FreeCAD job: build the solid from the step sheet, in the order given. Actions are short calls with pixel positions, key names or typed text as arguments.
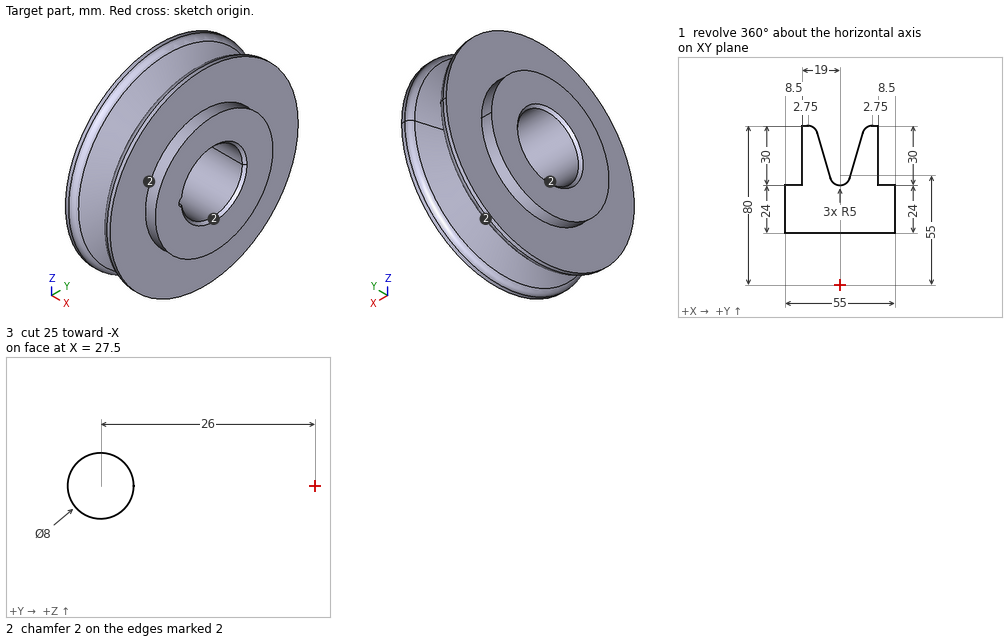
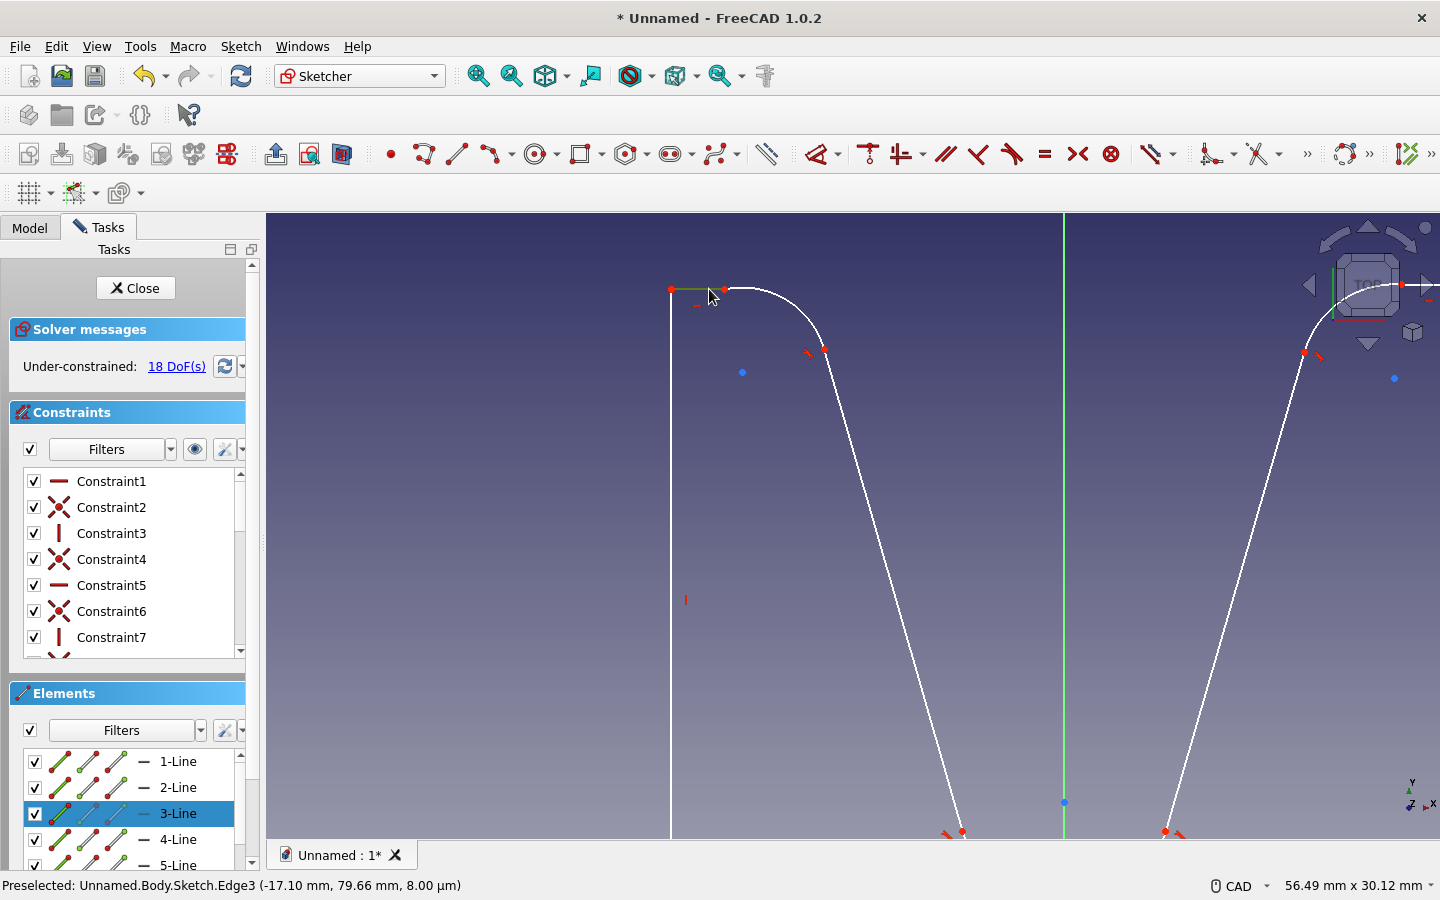
click(806, 316)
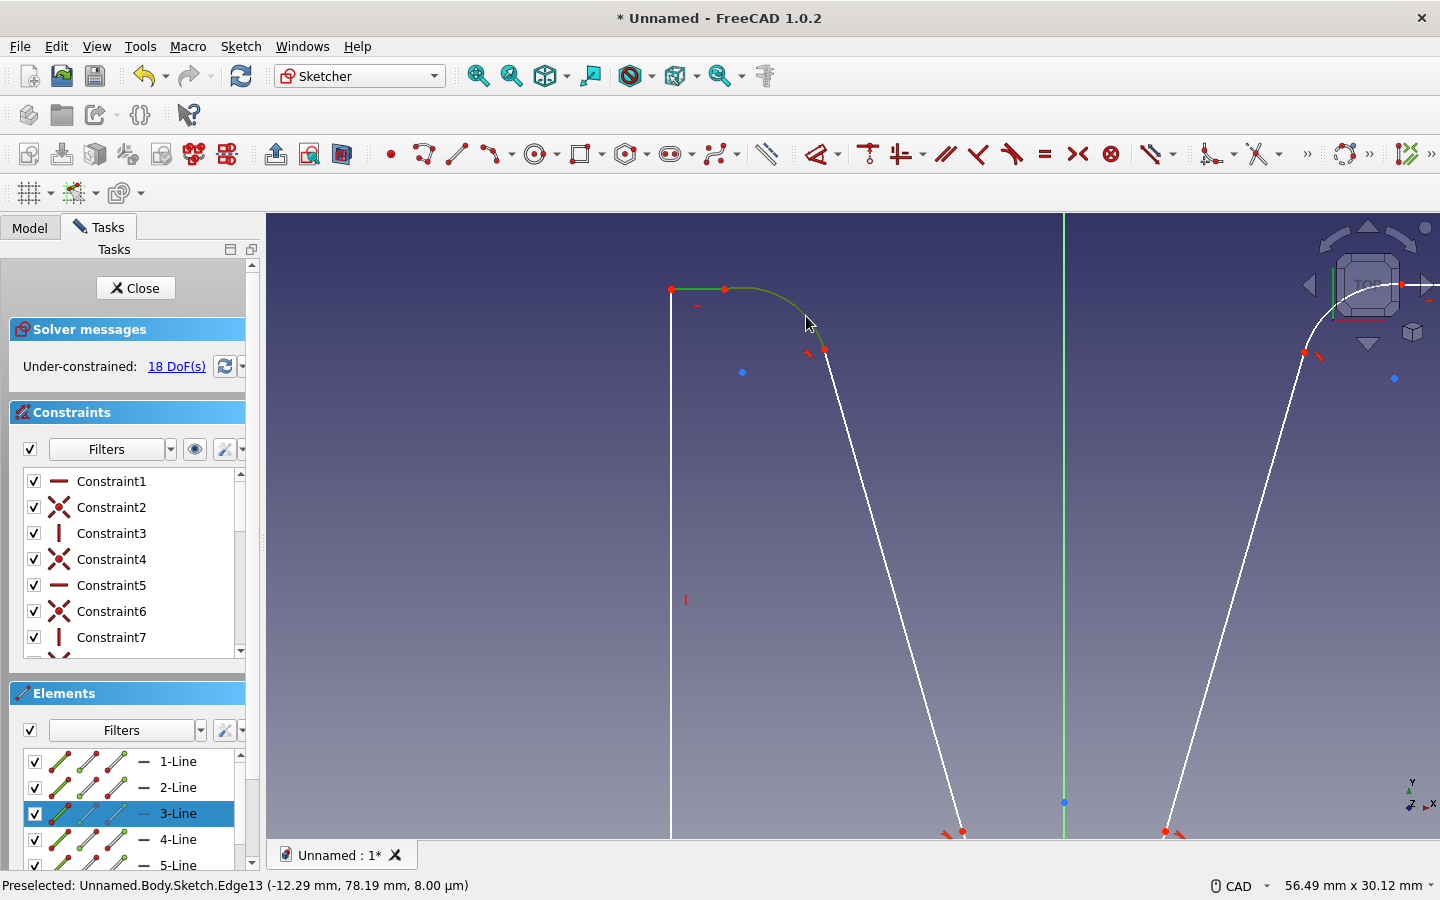
key(t)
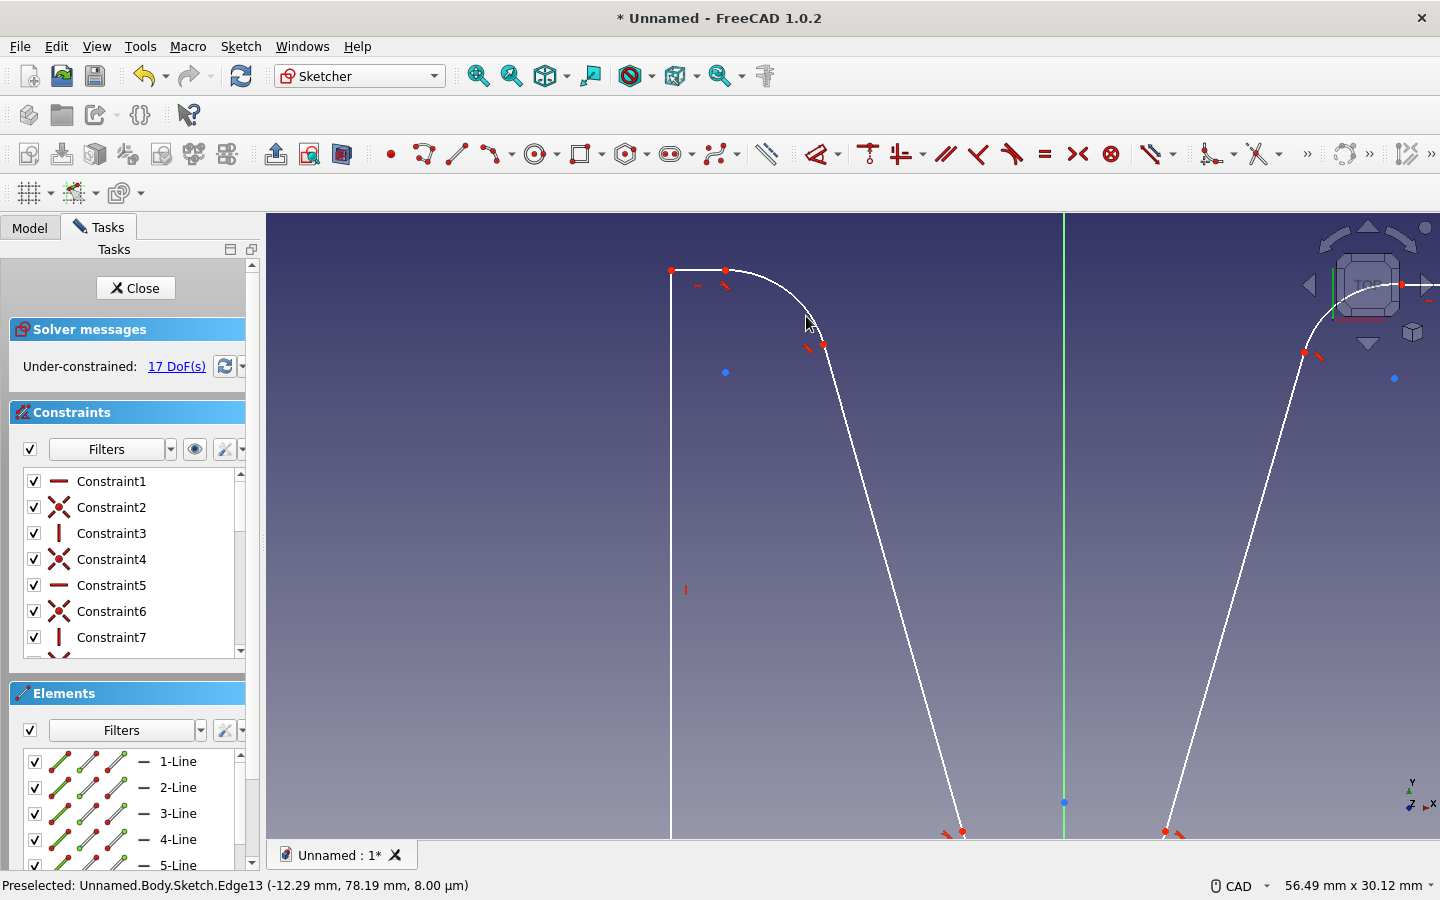
scroll(693, 334, down, 7)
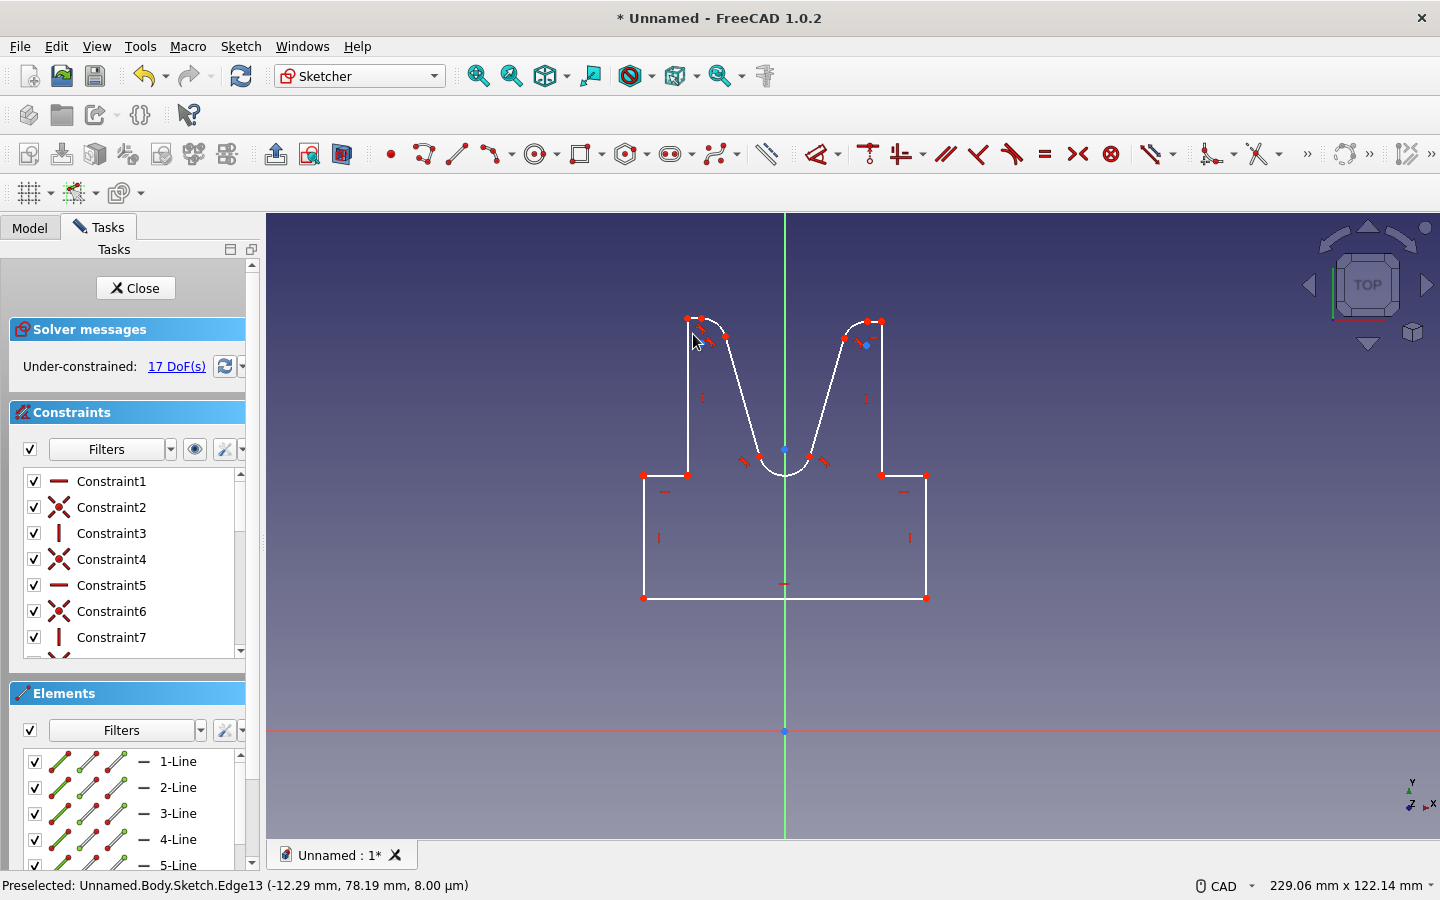
scroll(878, 322, up, 6)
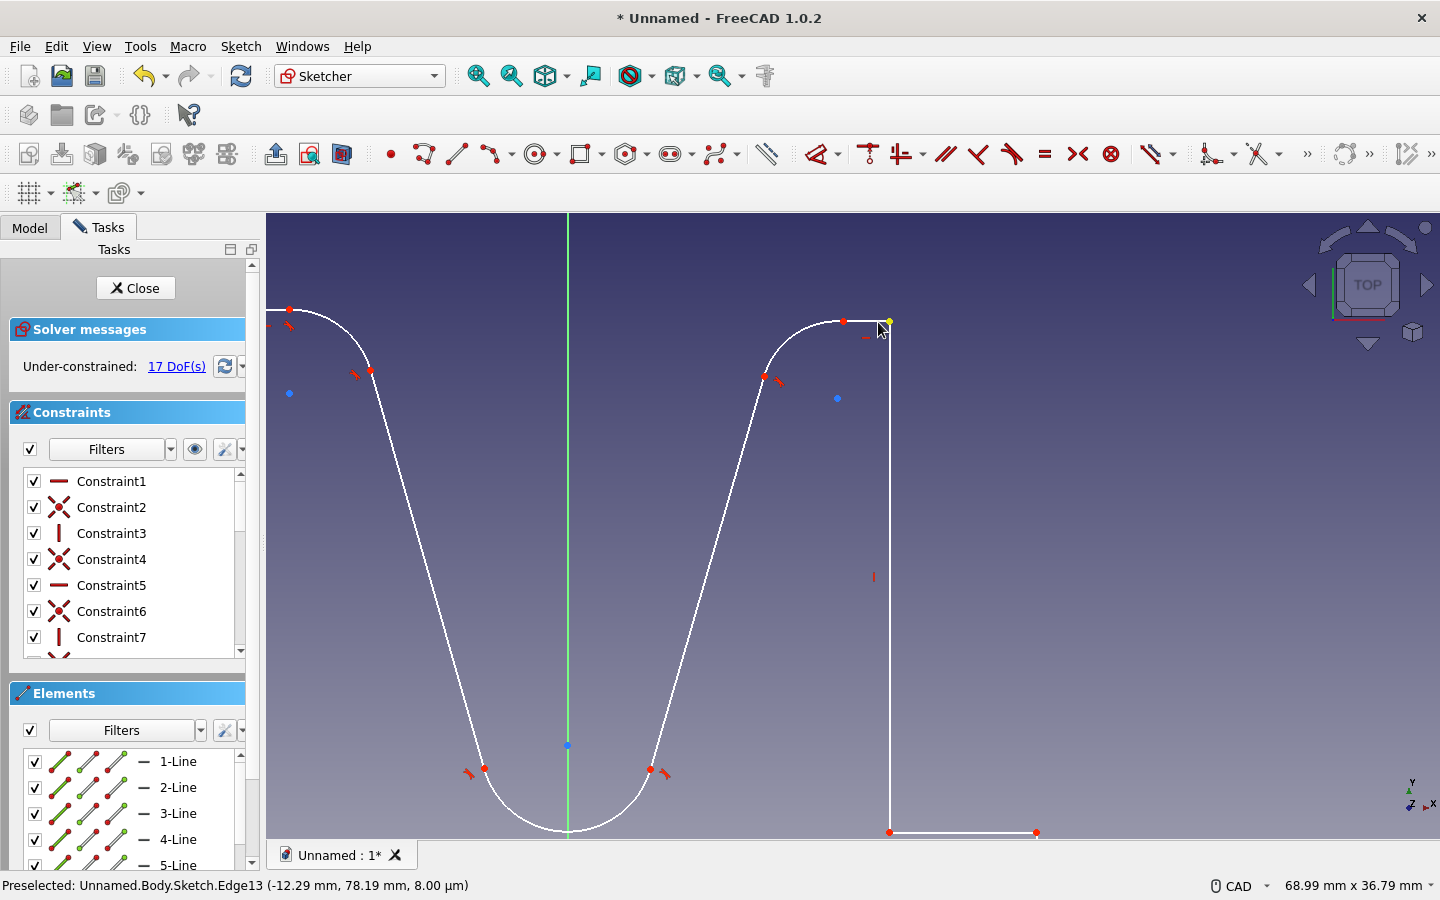
click(876, 321)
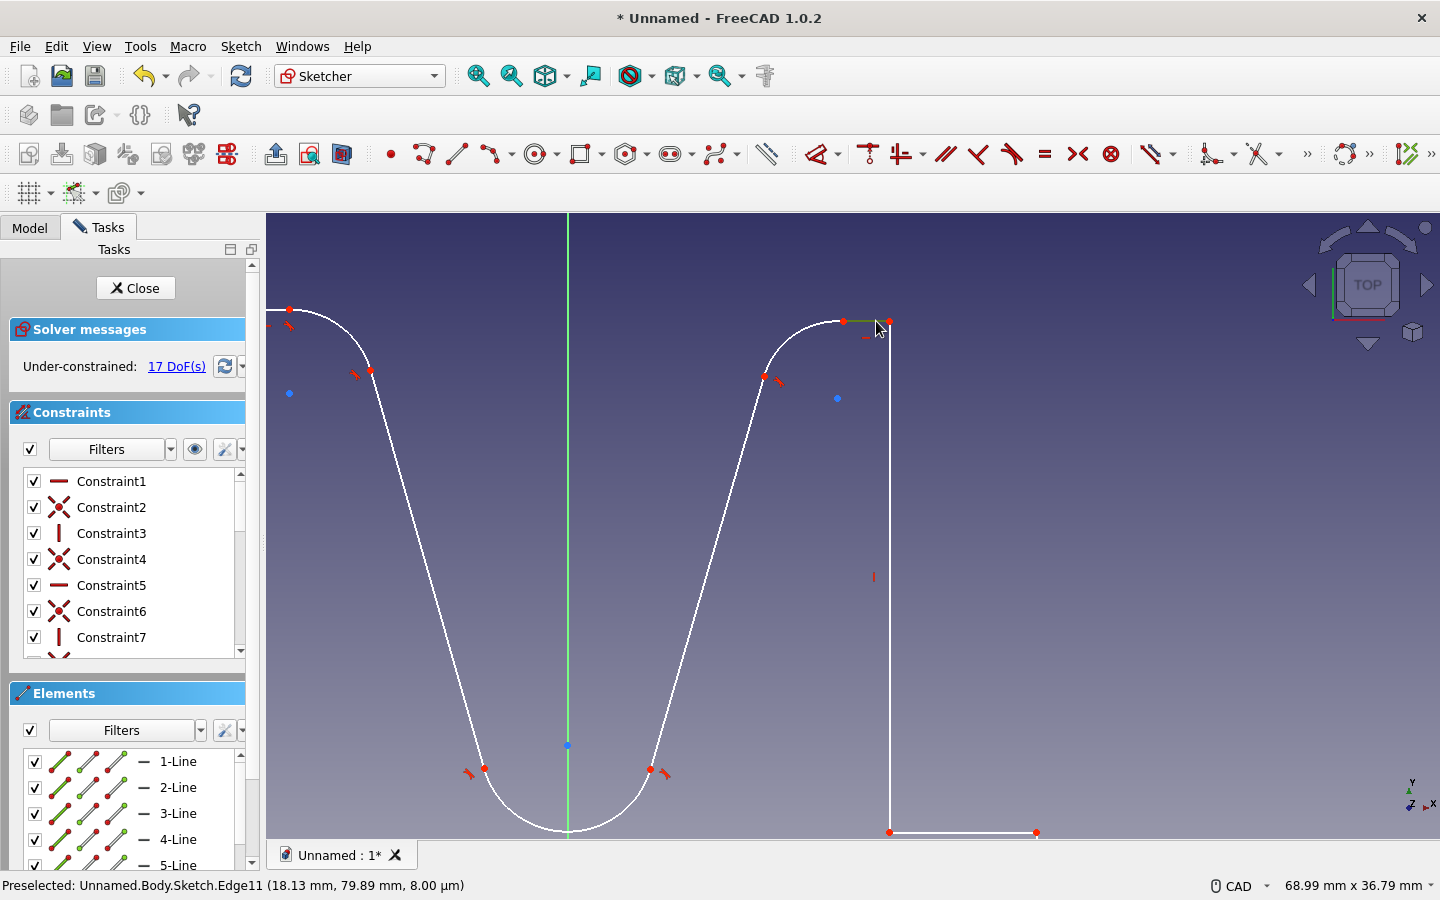
click(813, 326)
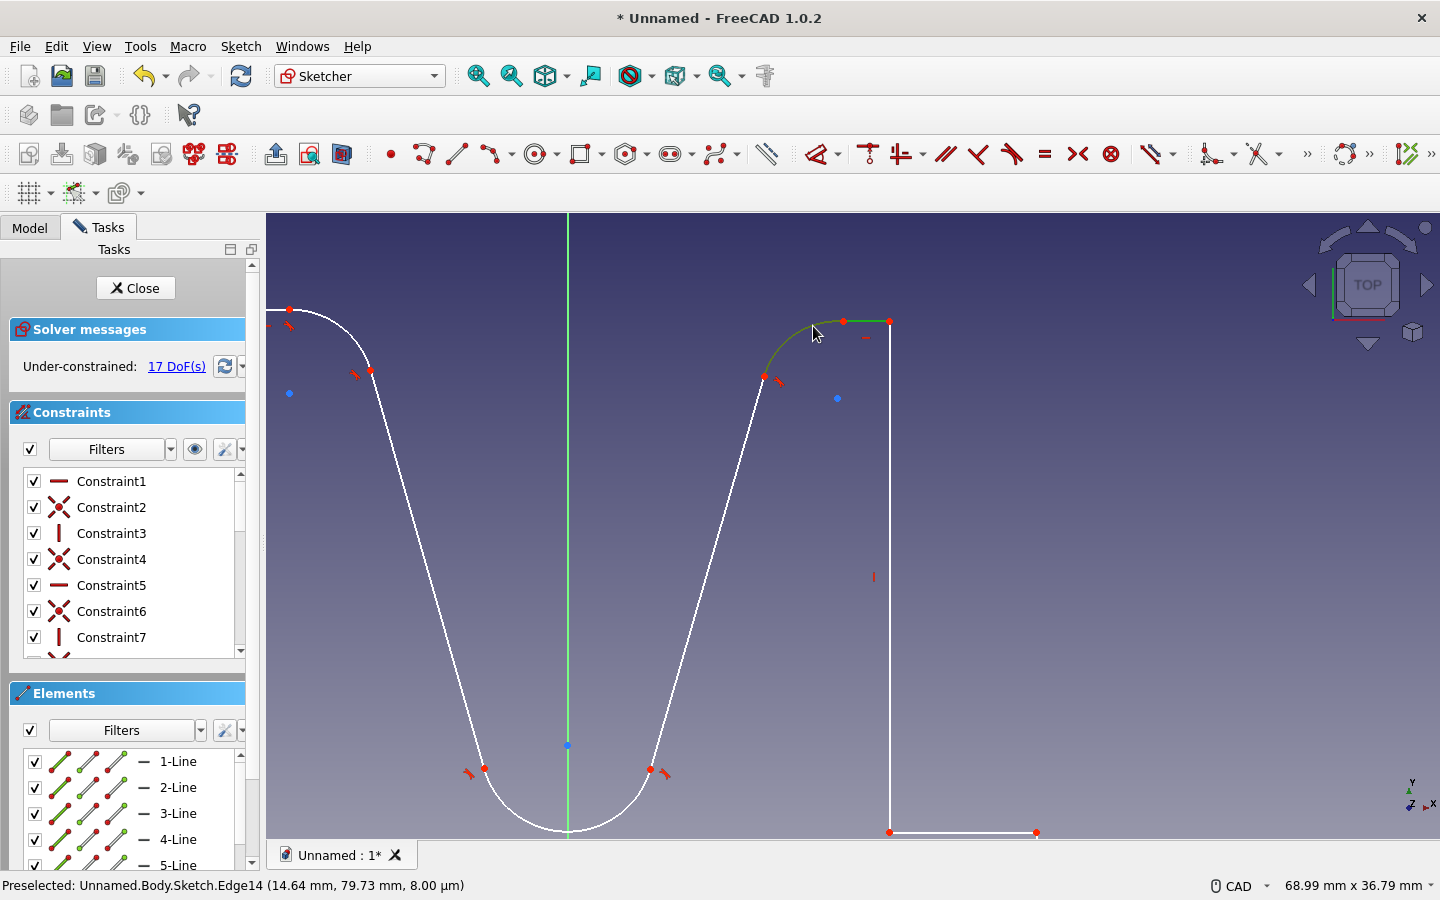
key(t)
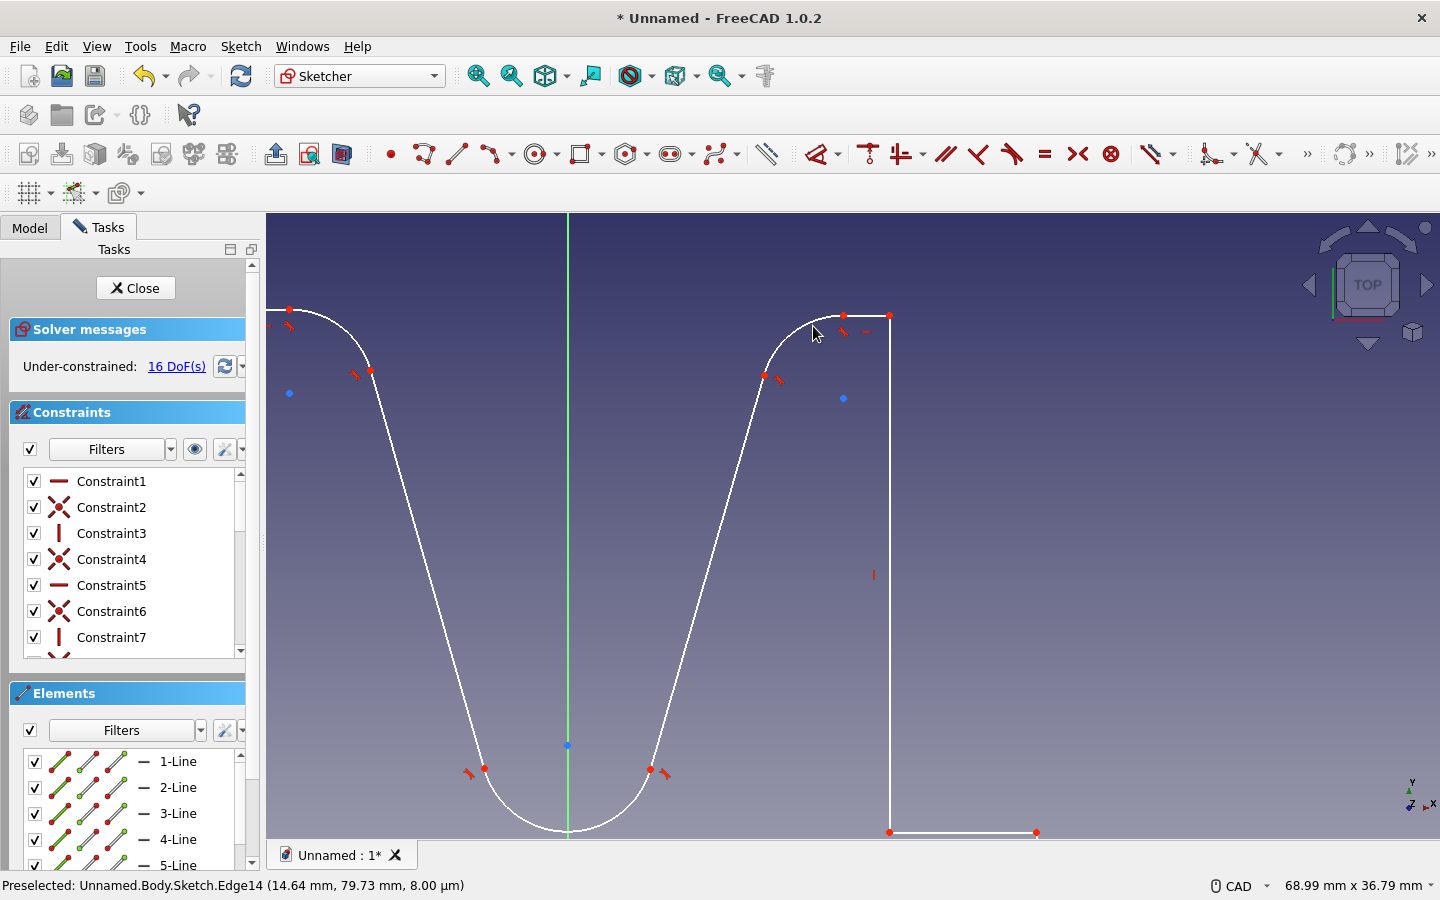
scroll(878, 322, down, 6)